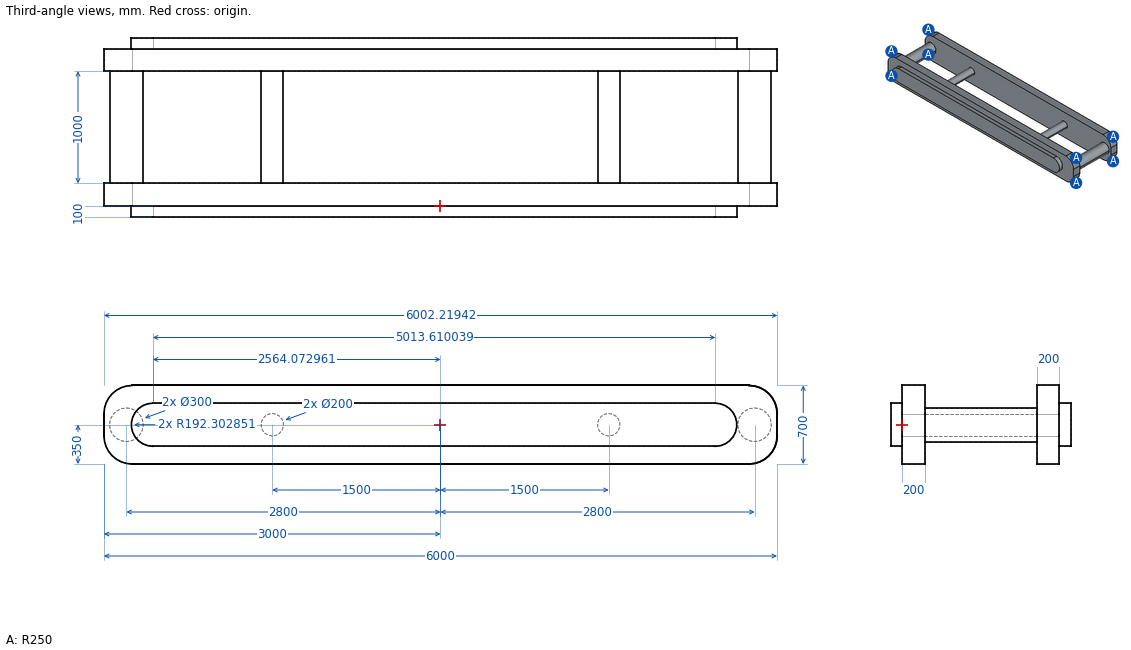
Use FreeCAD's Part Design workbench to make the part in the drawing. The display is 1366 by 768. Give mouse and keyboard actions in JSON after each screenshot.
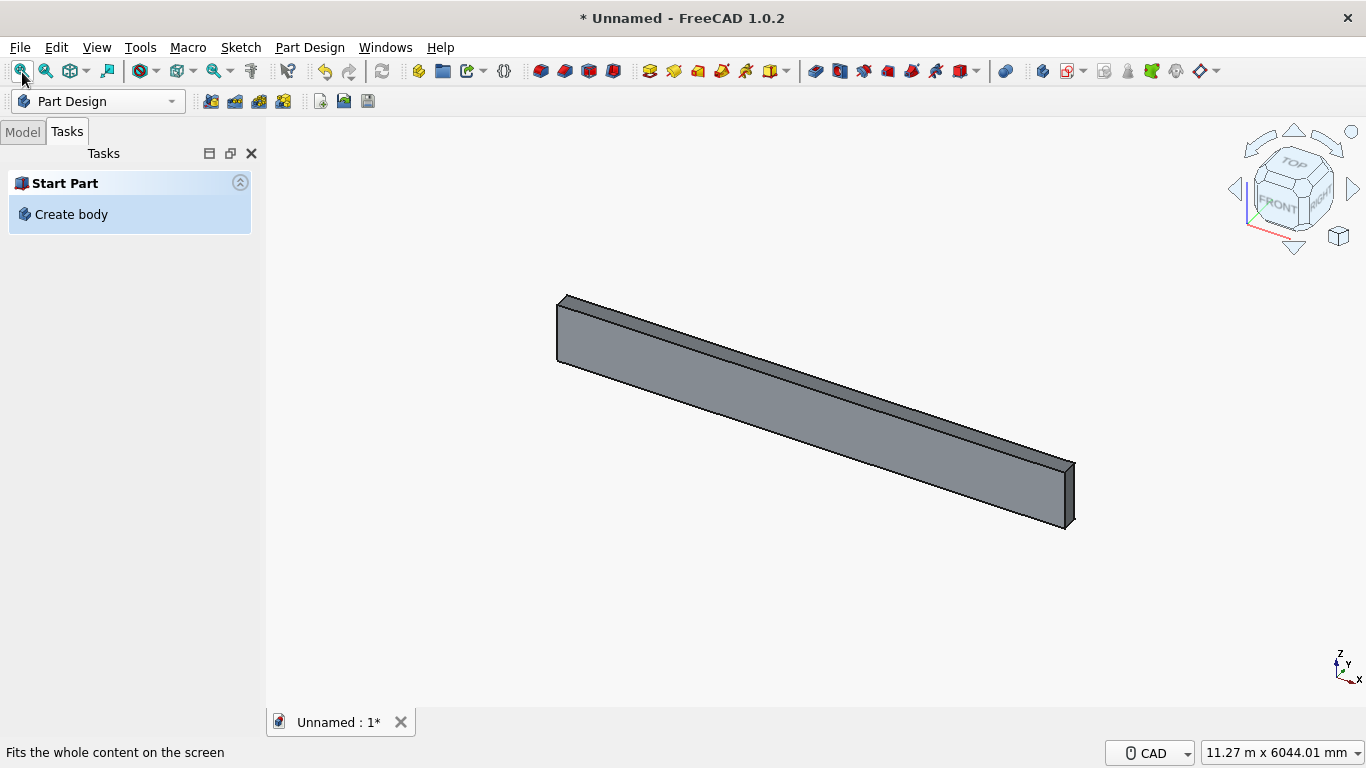
{"action": "key", "text": "4"}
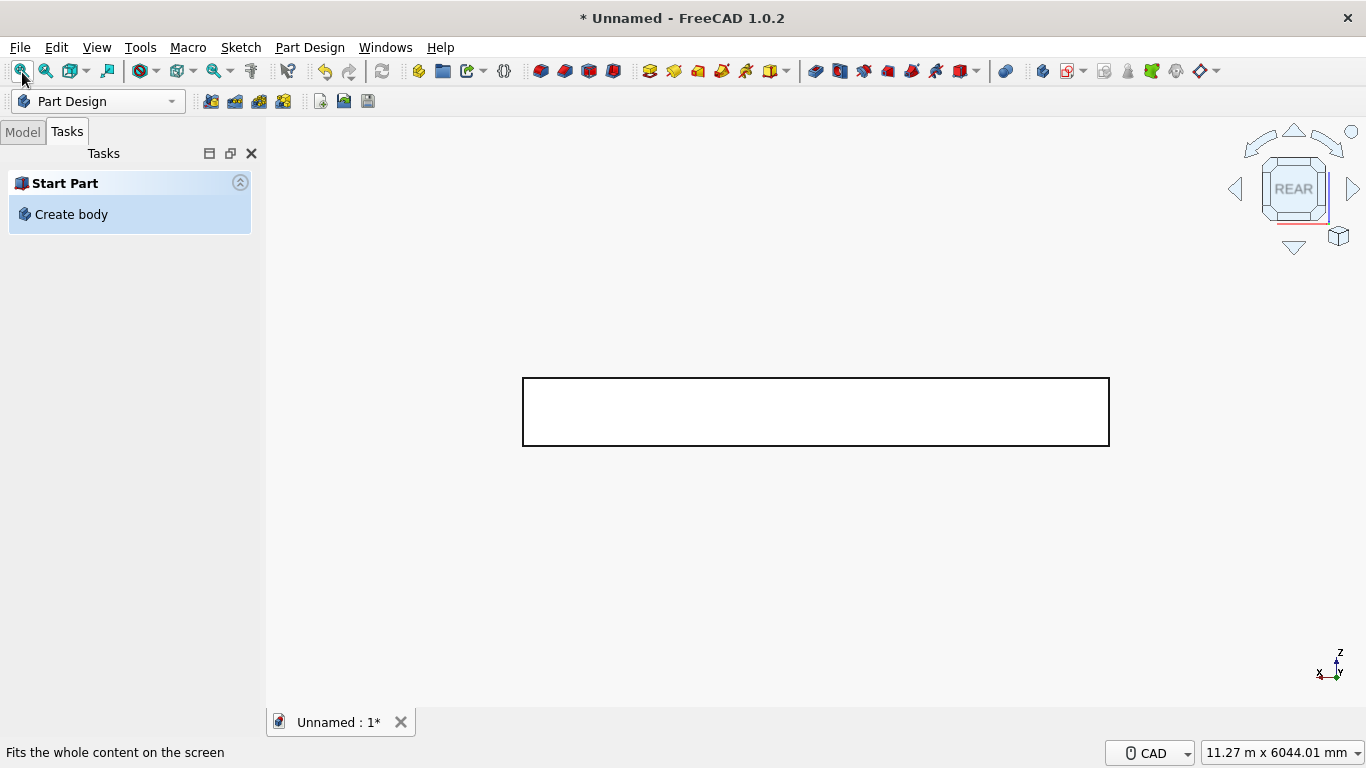
{"action": "left_click", "coordinate": [565, 411]}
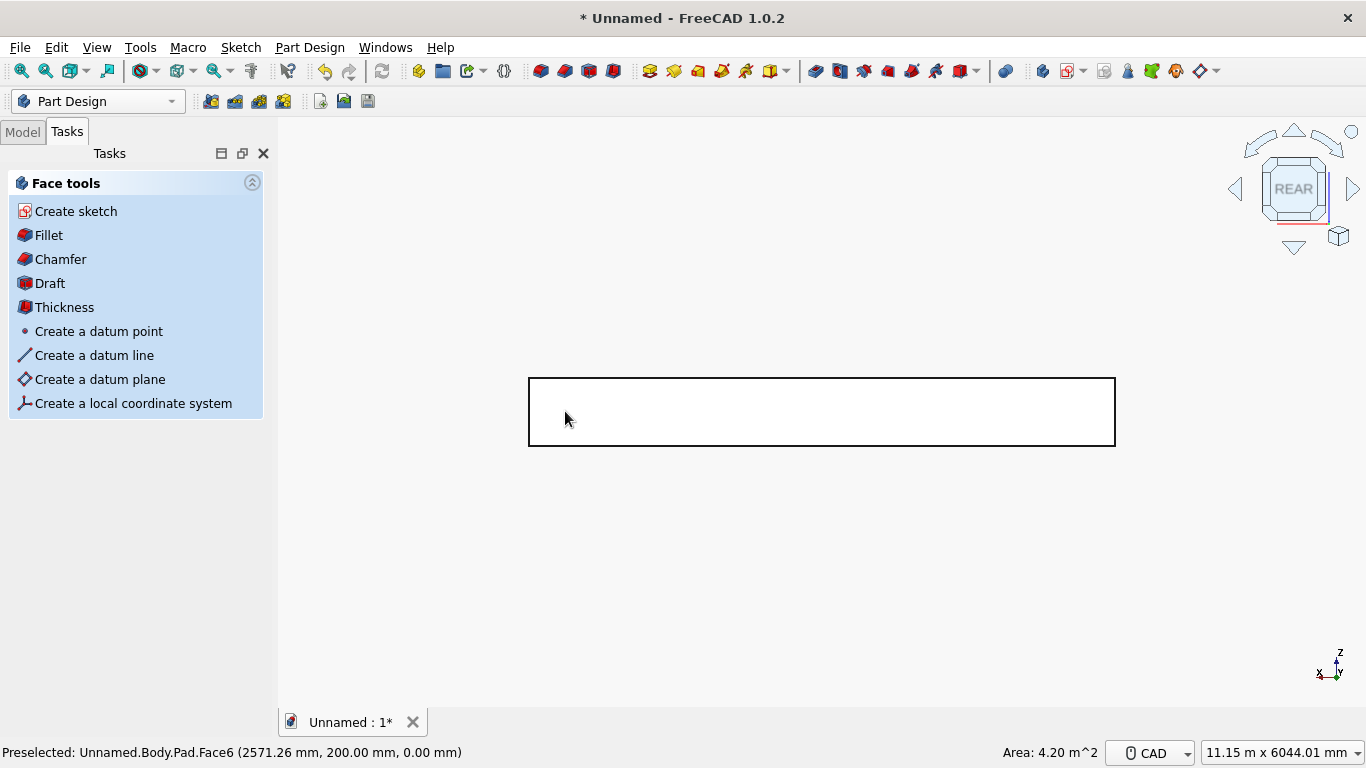
{"action": "left_click", "coordinate": [1068, 72]}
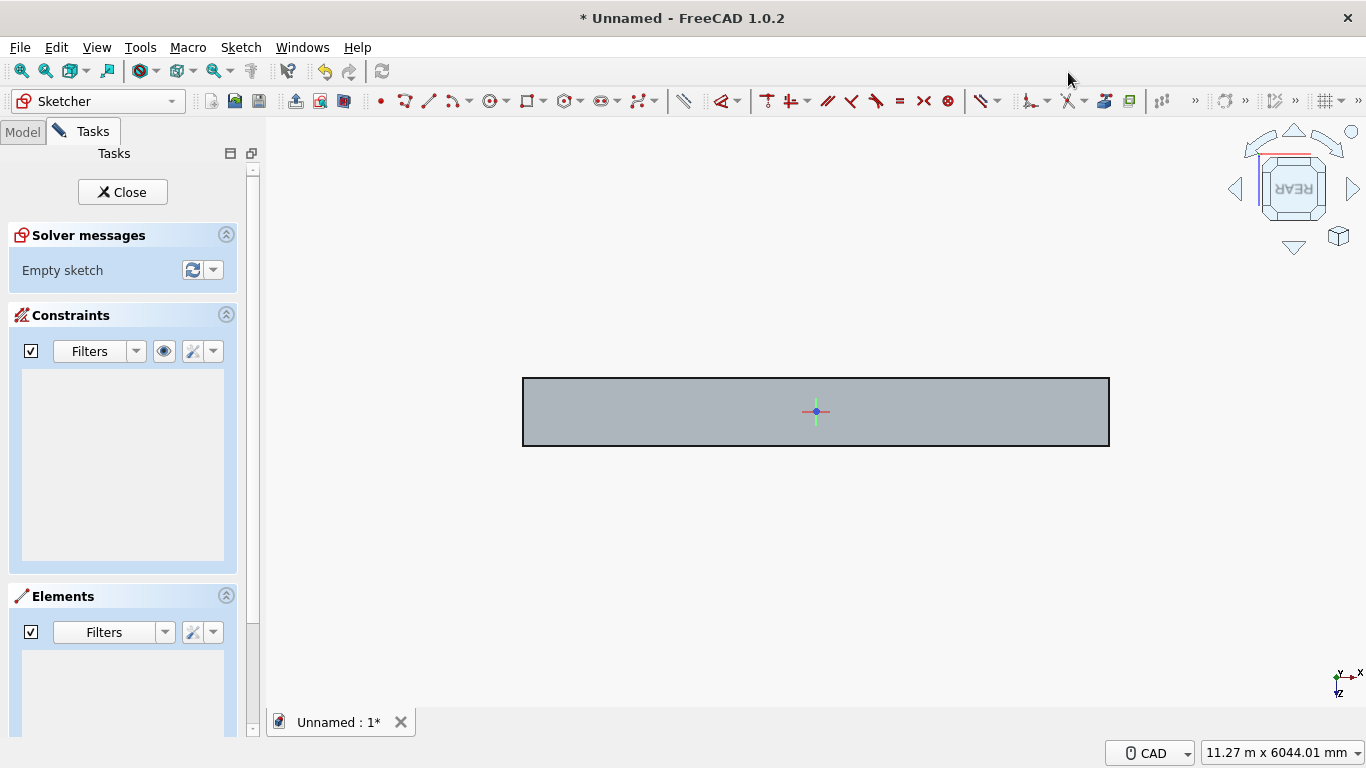
{"action": "key", "text": "g c"}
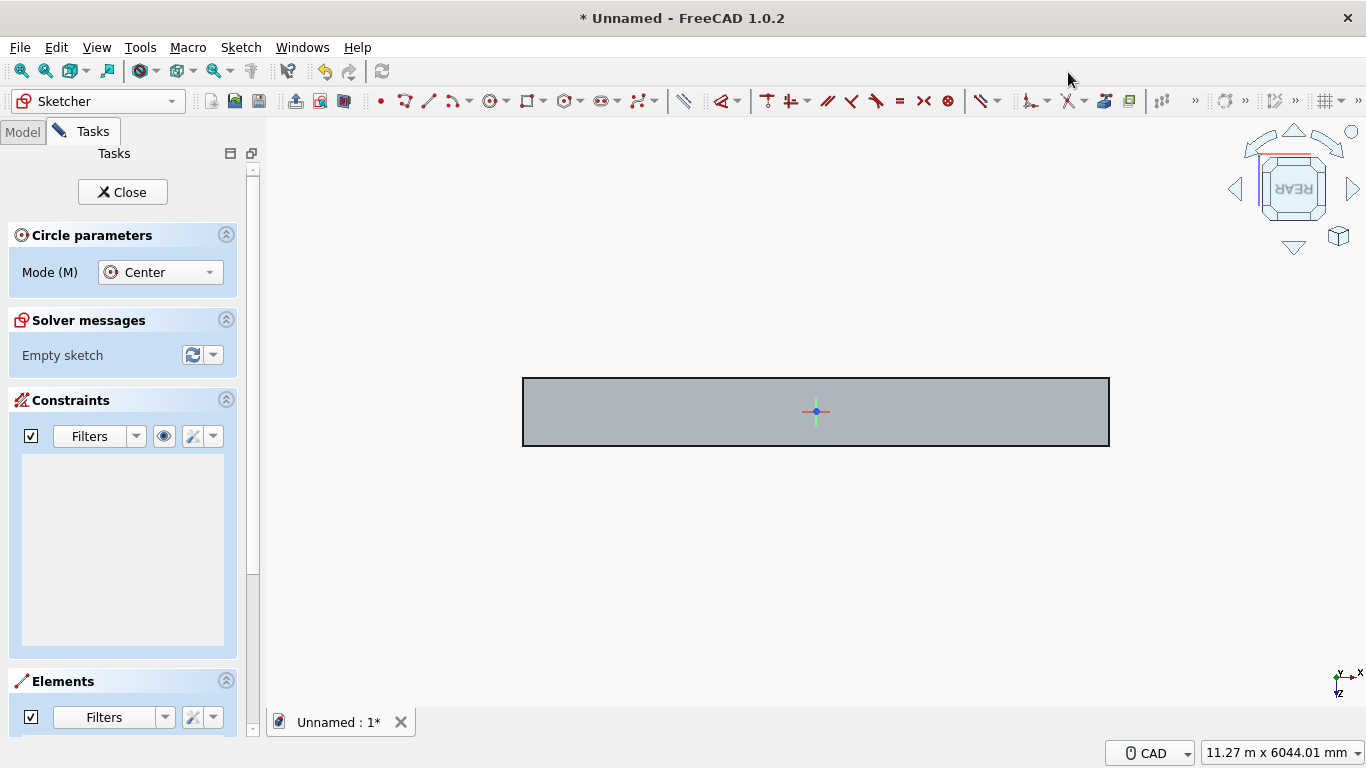
{"action": "scroll", "coordinate": [543, 412], "scroll_direction": "up", "scroll_amount": 3}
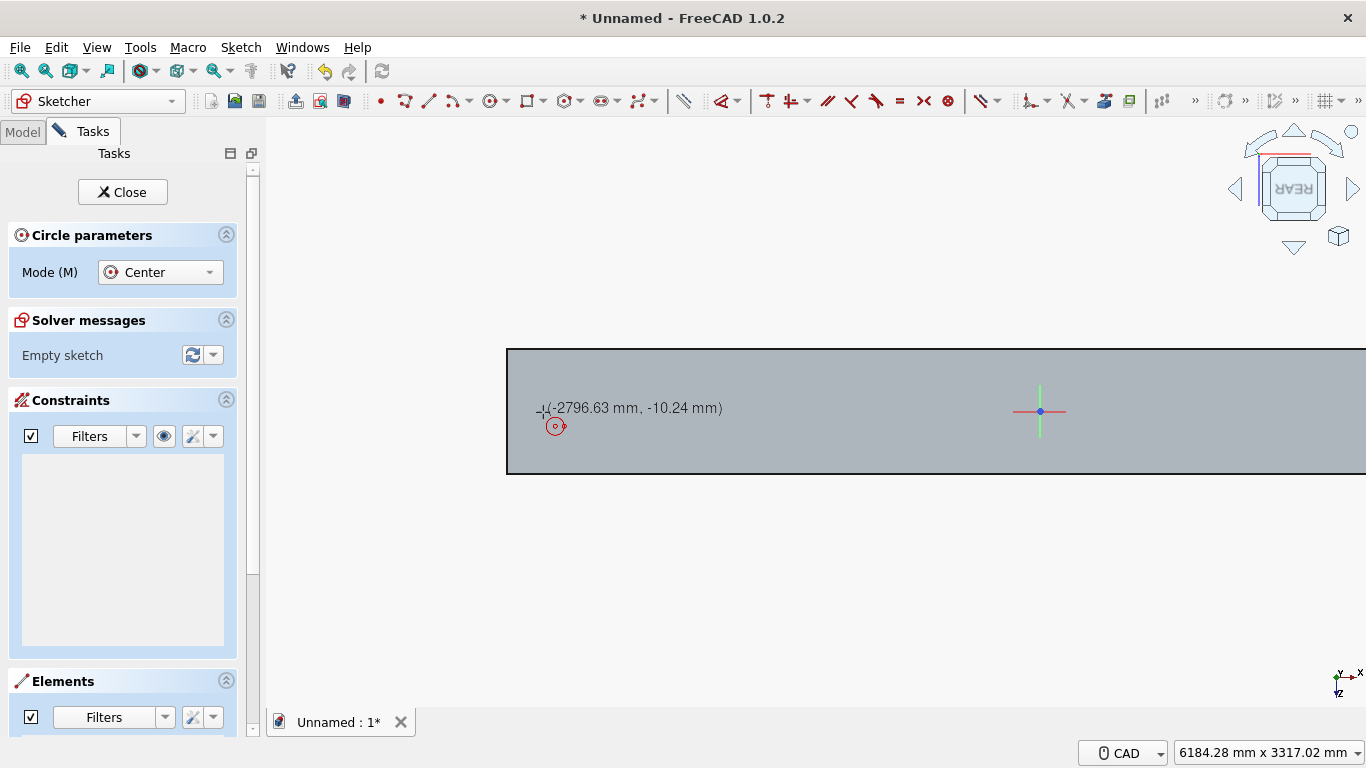
{"action": "left_click", "coordinate": [542, 412]}
{"action": "left_click", "coordinate": [561, 393]}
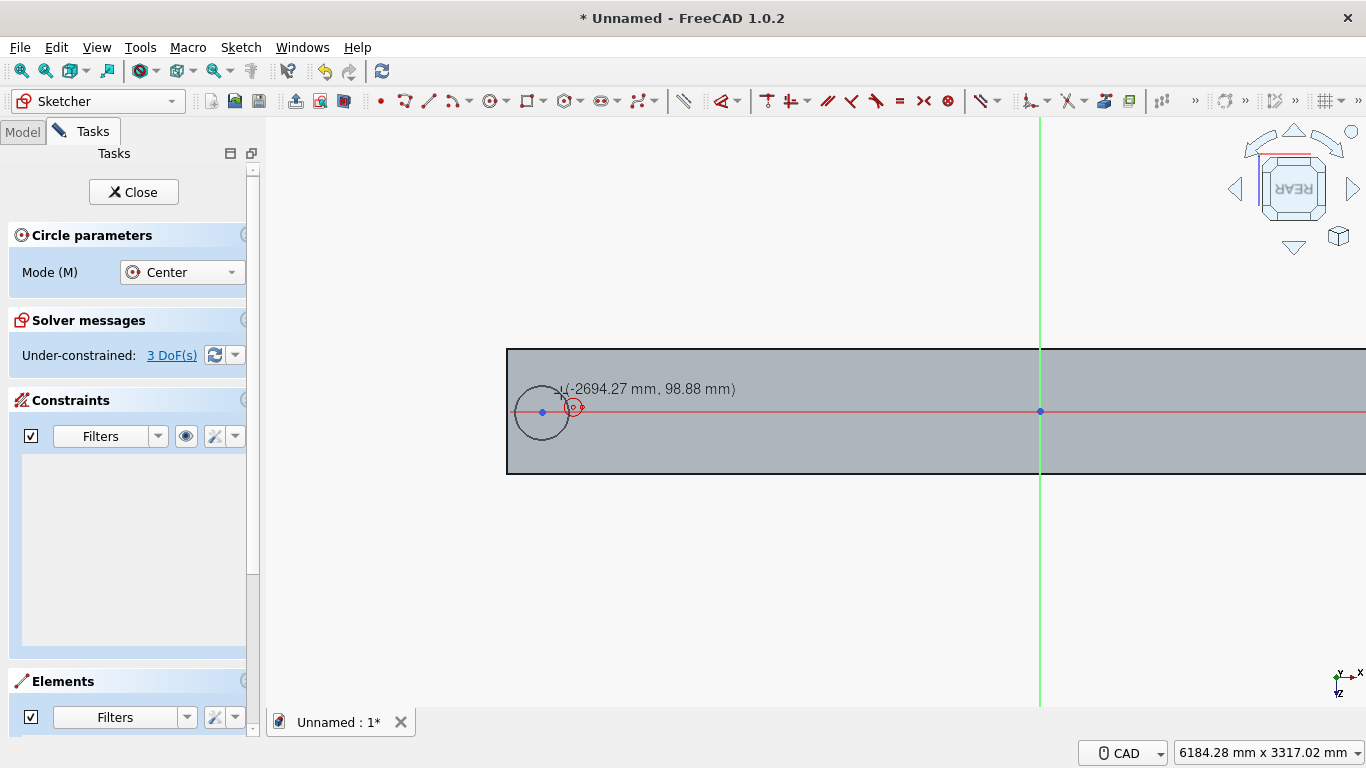
{"action": "scroll", "coordinate": [294, 413], "scroll_direction": "down", "scroll_amount": 2}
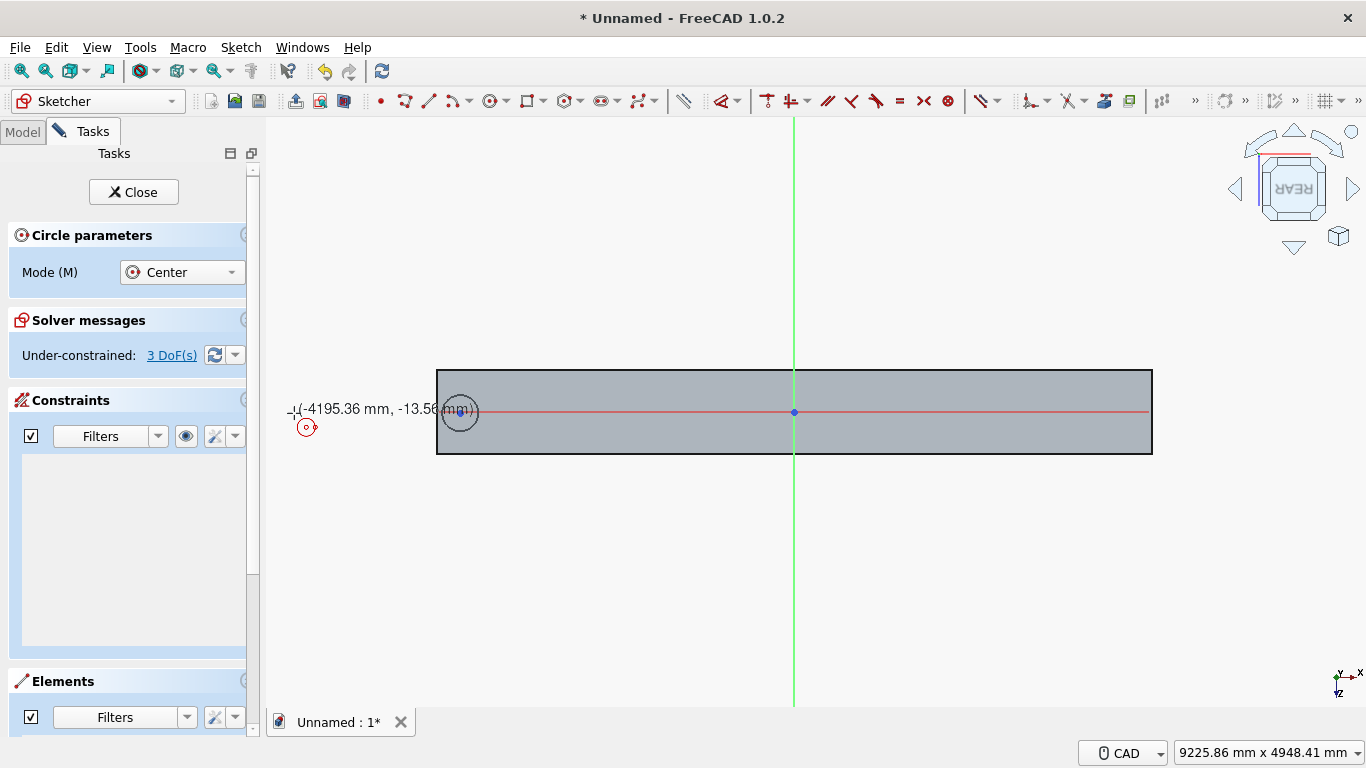
{"action": "scroll", "coordinate": [1128, 412], "scroll_direction": "up", "scroll_amount": 2}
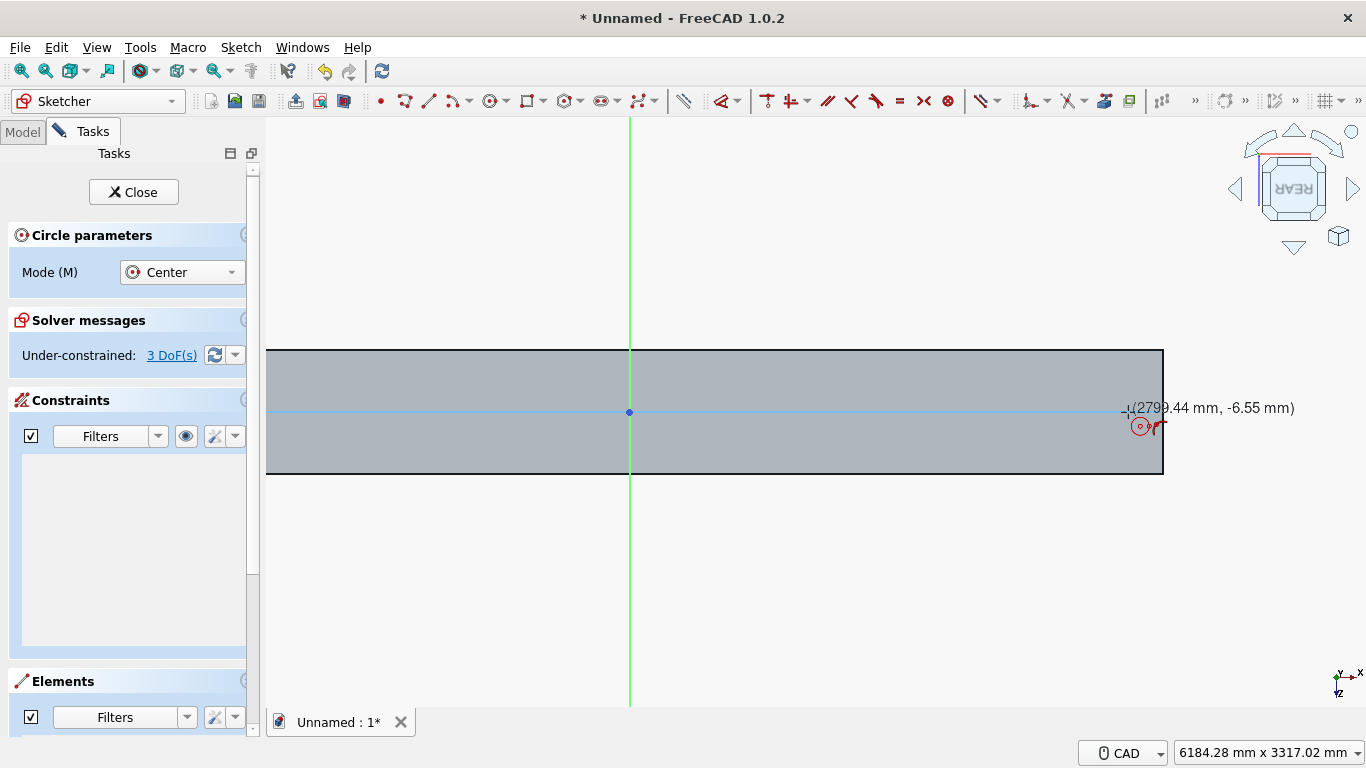
{"action": "left_click", "coordinate": [1128, 412]}
{"action": "left_click", "coordinate": [1147, 393]}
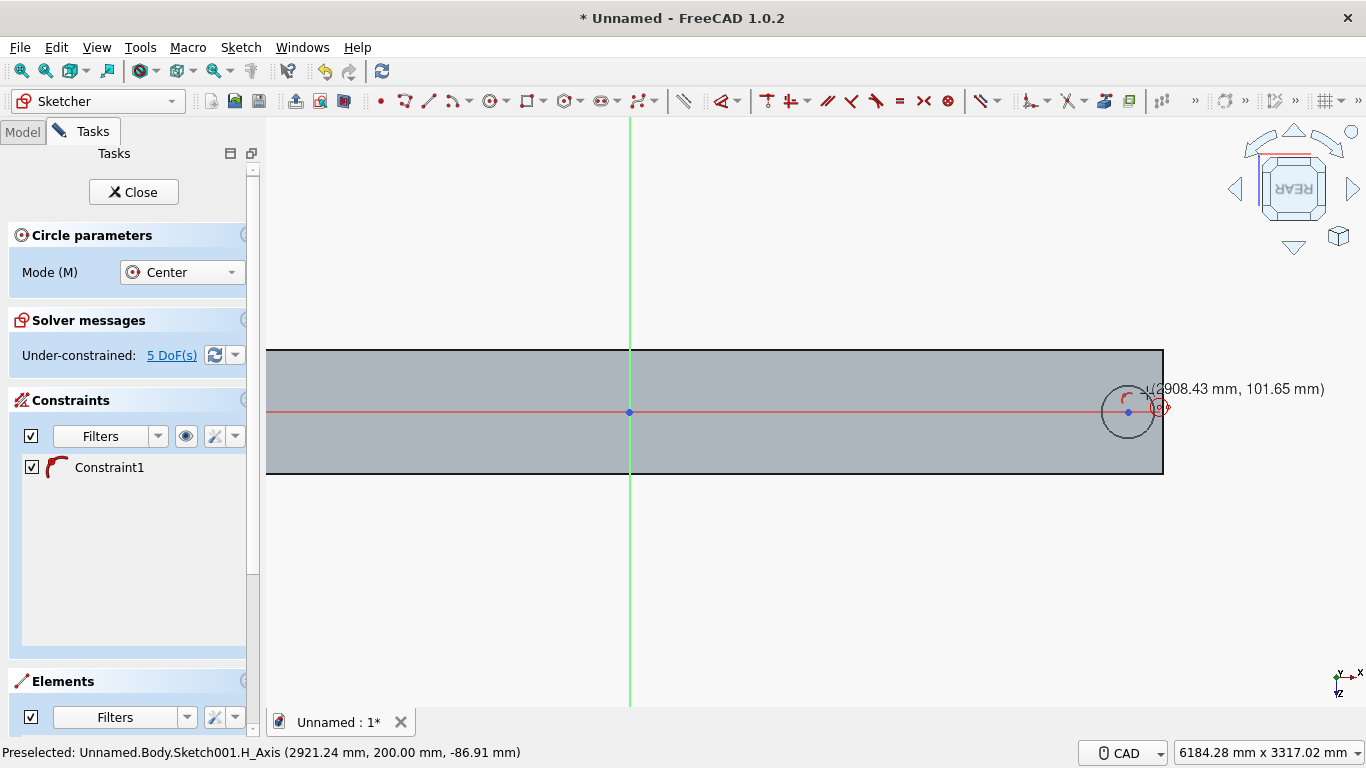
{"action": "scroll", "coordinate": [363, 412], "scroll_direction": "up", "scroll_amount": 2}